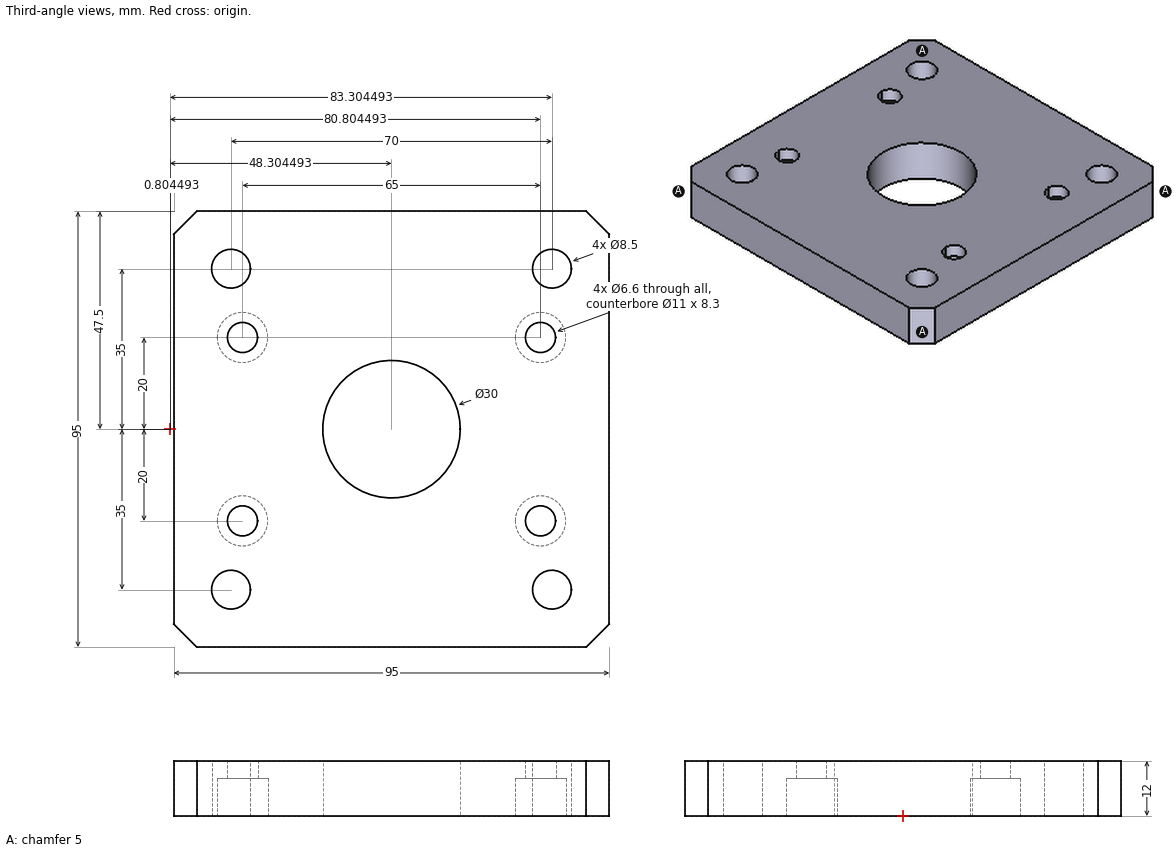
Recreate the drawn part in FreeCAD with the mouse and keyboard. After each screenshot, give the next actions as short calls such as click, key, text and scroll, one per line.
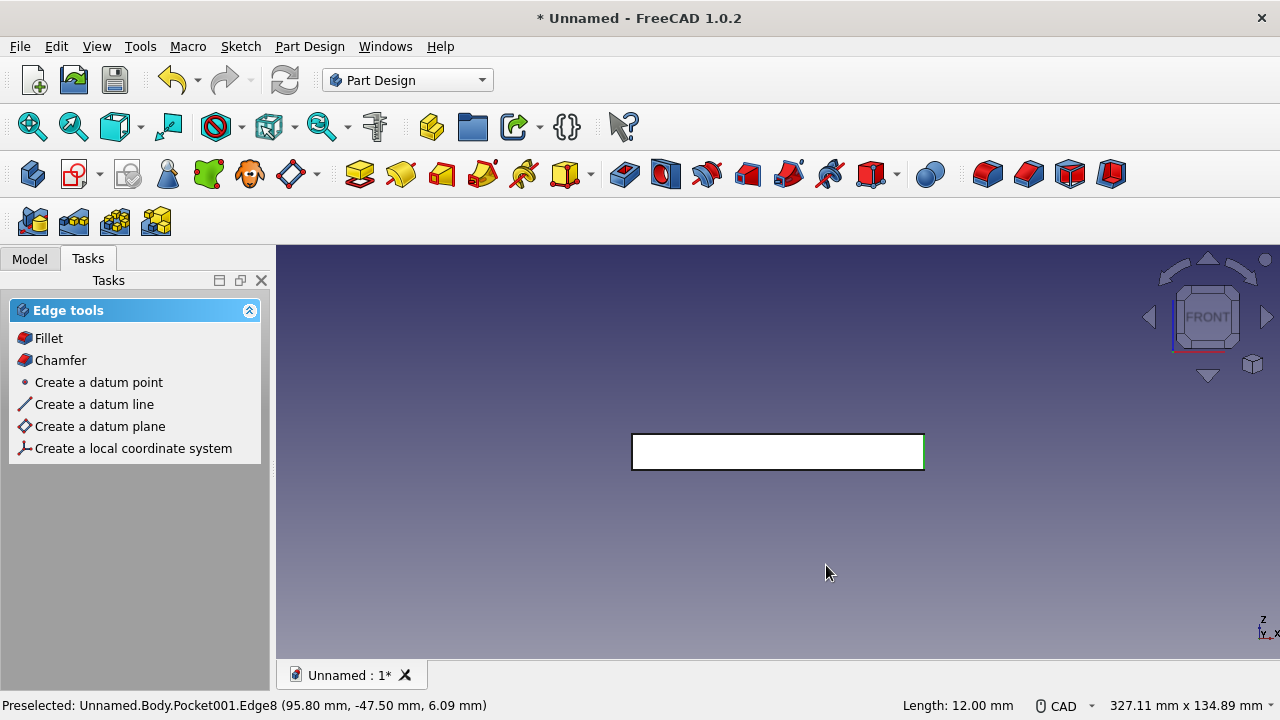
click(33, 128)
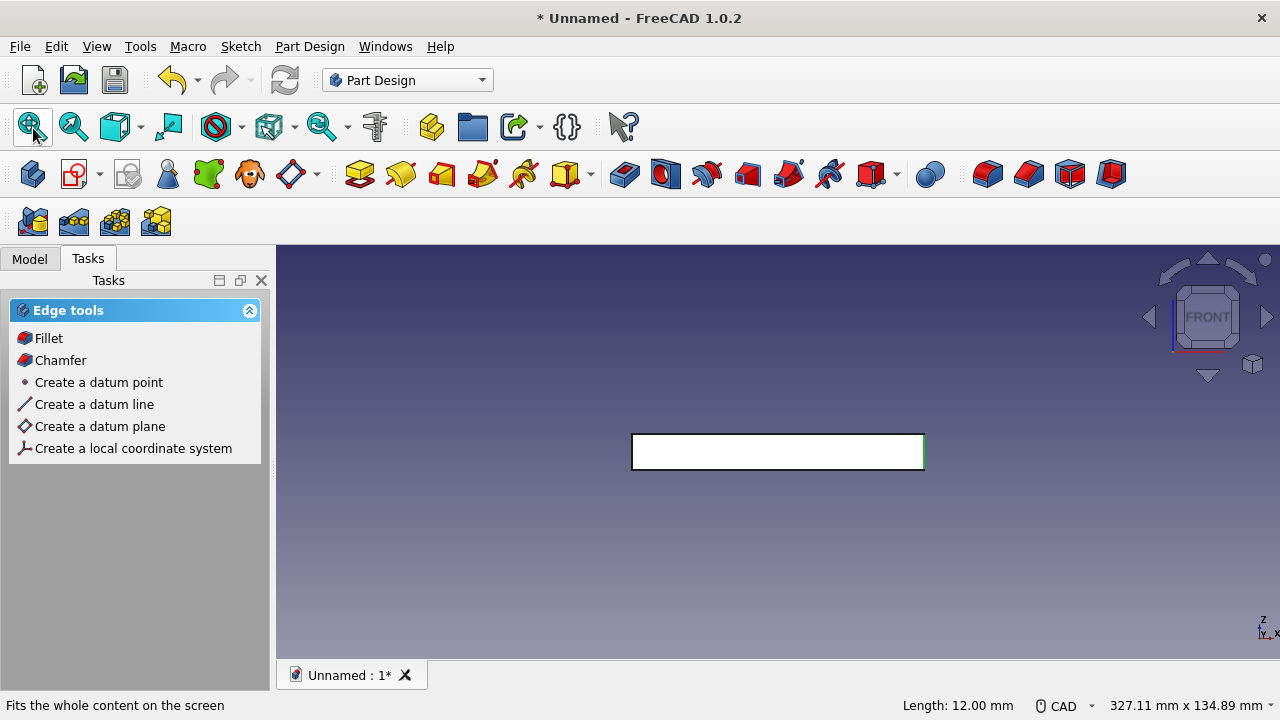
click(632, 451, ctrl)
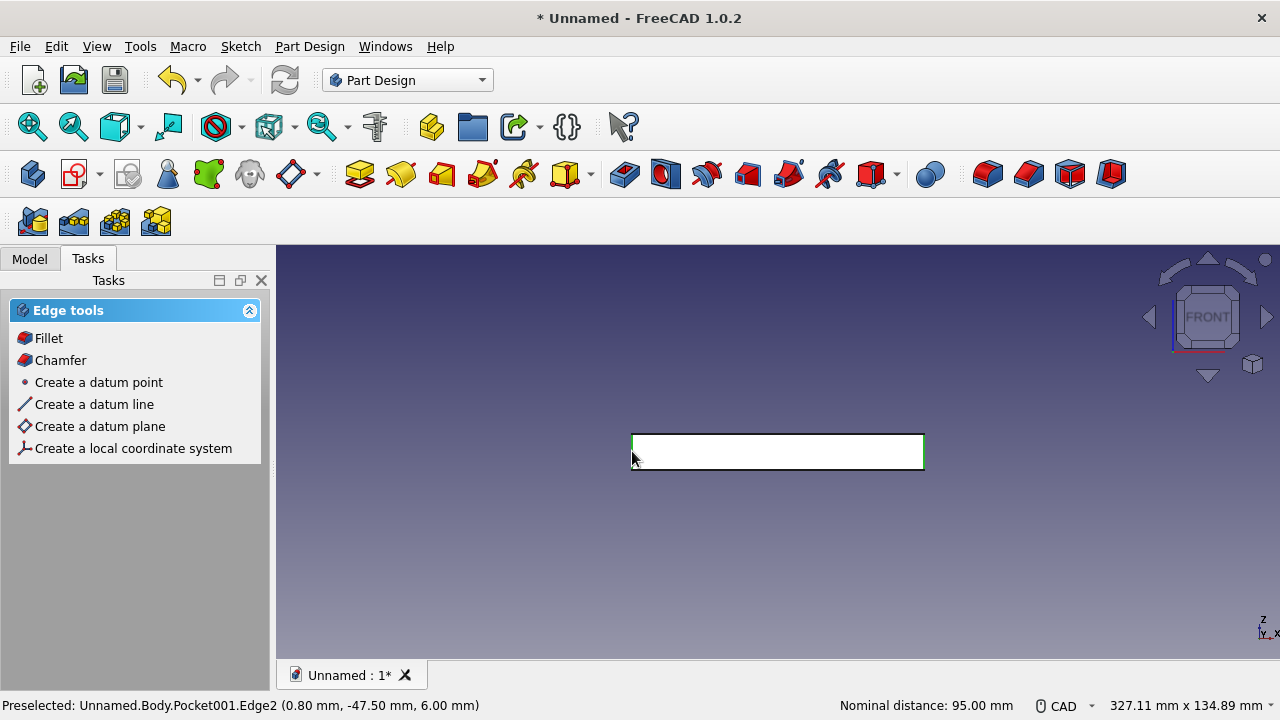
key(3)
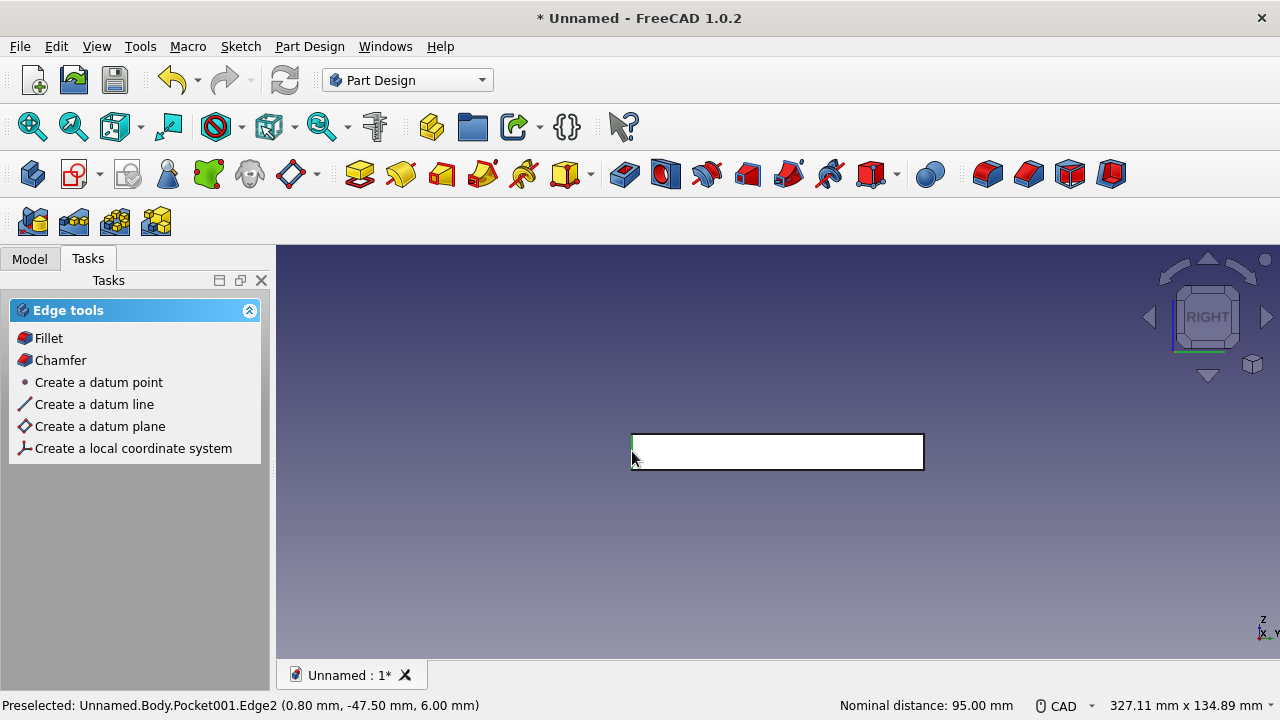
key(v)
key(f)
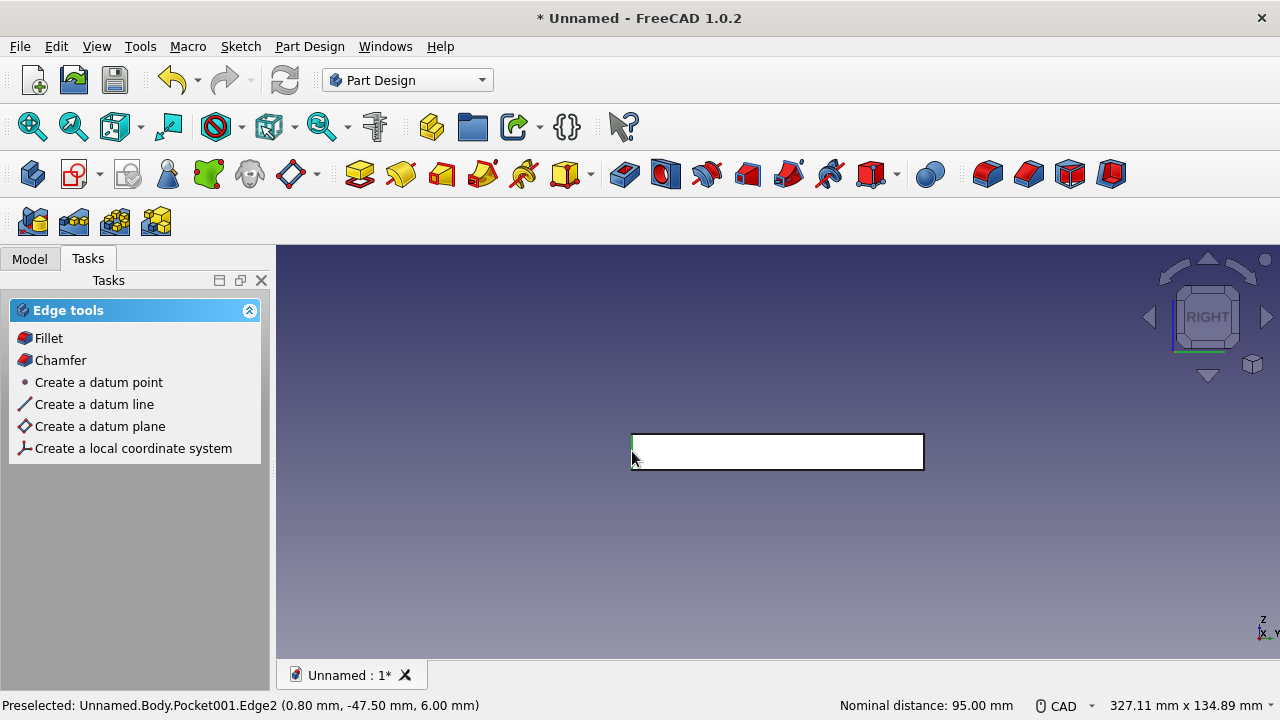
click(924, 451, ctrl)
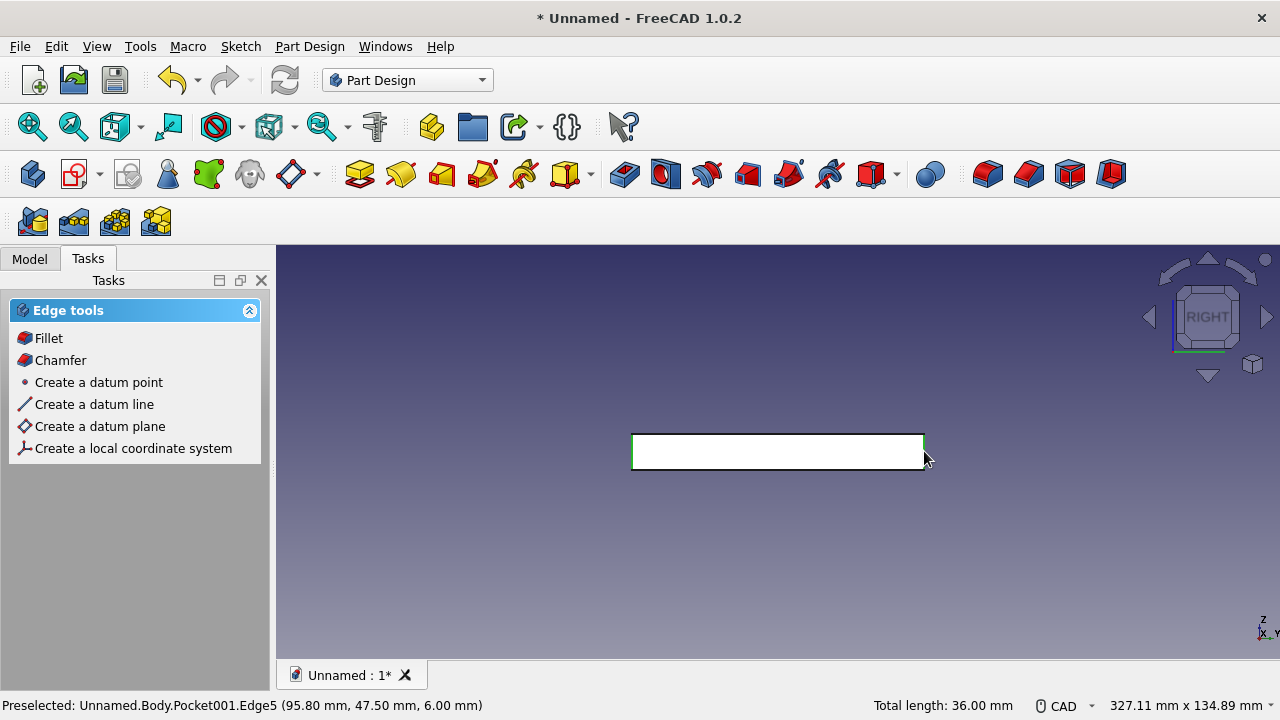
key(5)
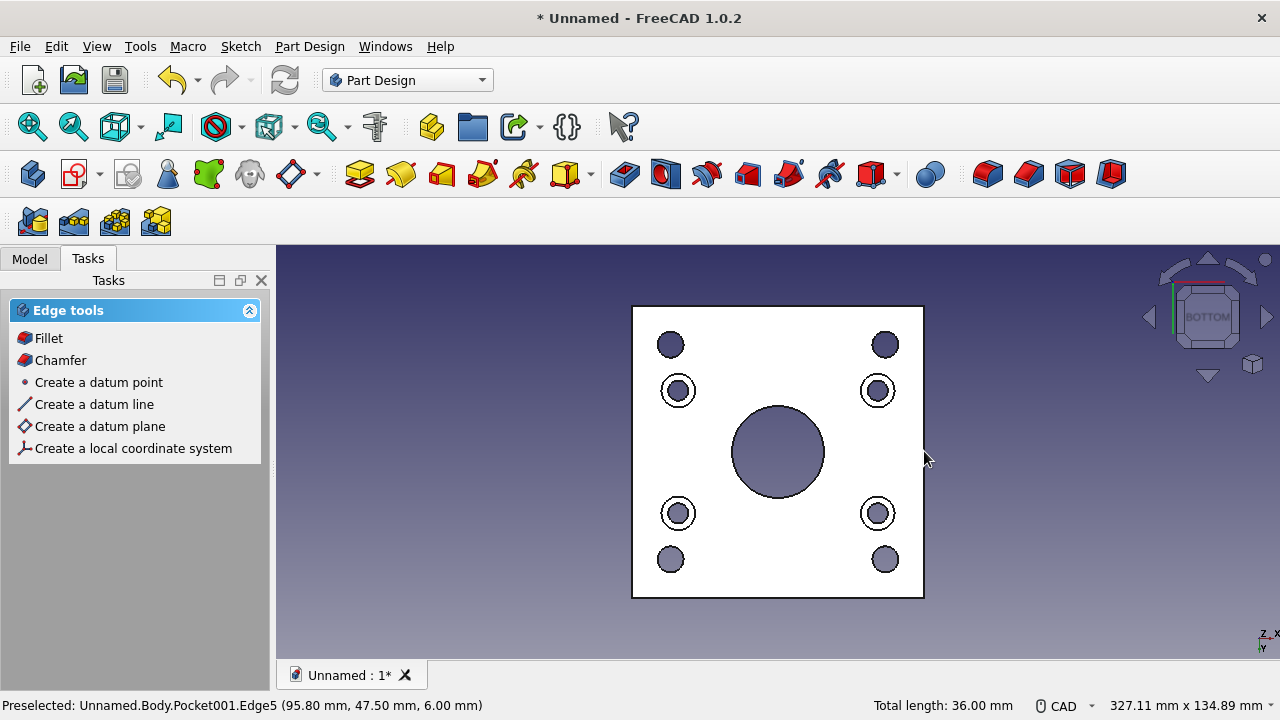
key(4)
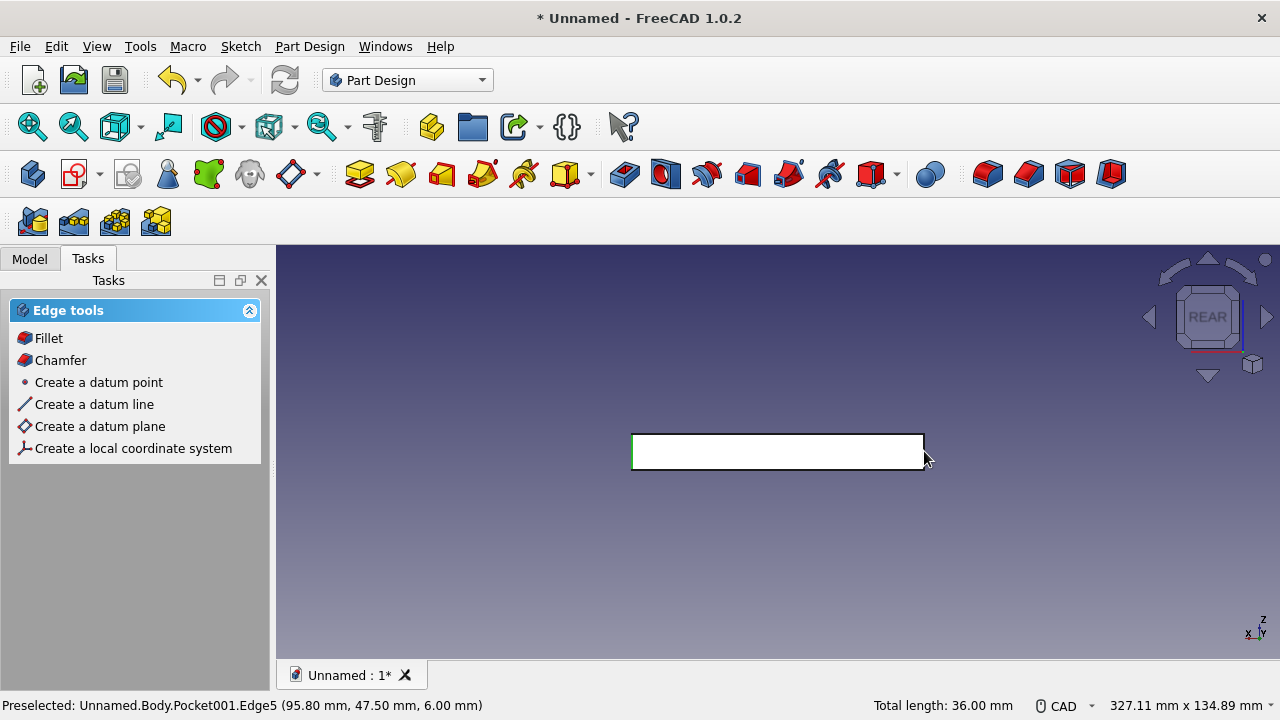
key(v)
key(f)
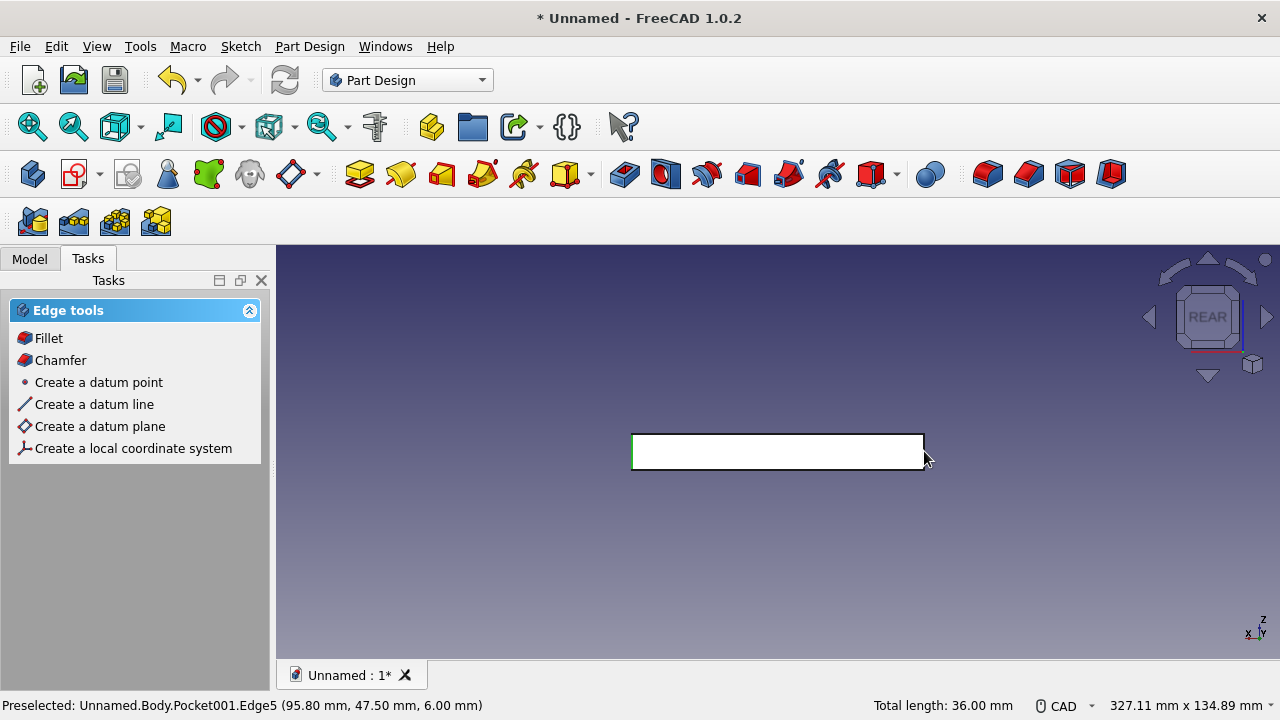
click(924, 451, ctrl)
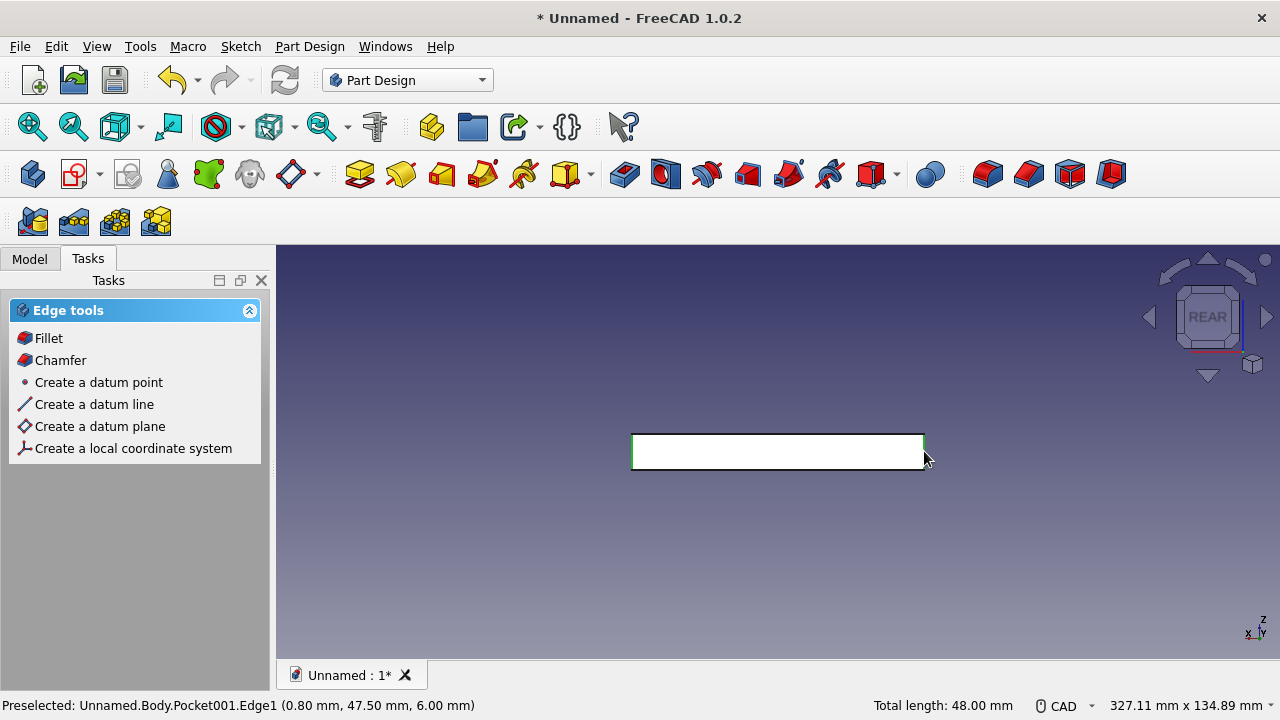
click(1029, 174)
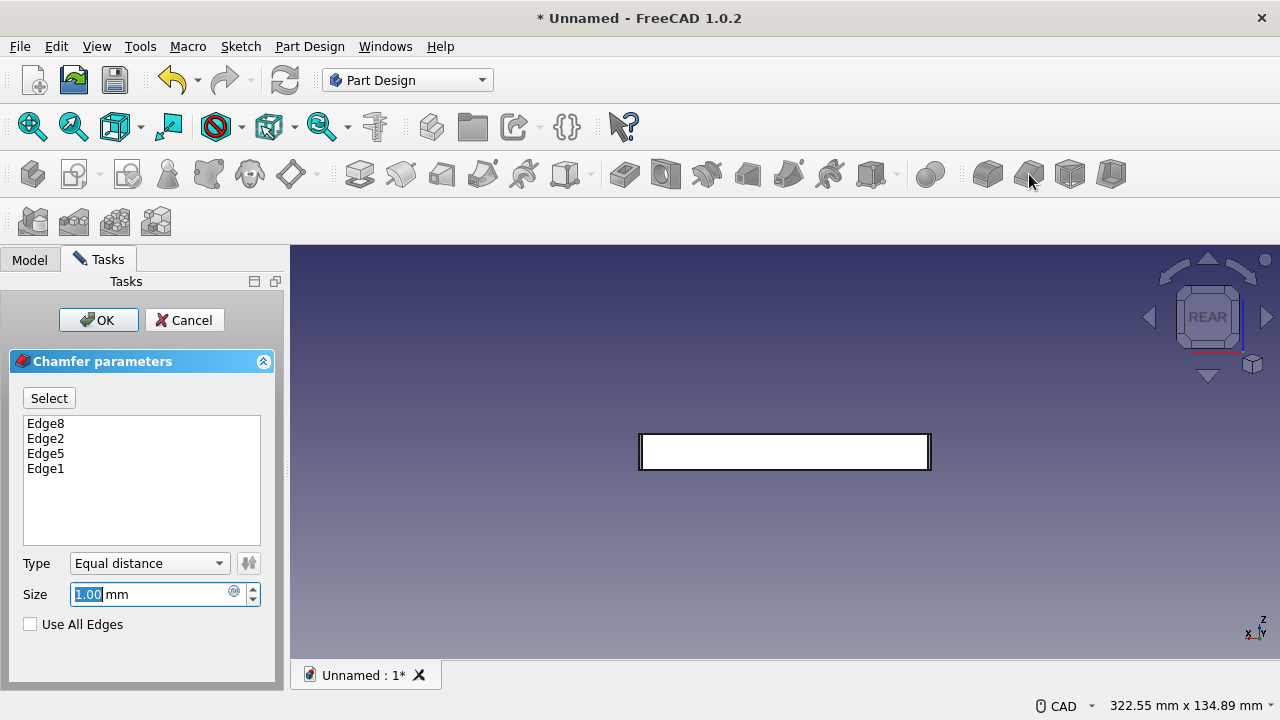
text(5)
key(Tab)